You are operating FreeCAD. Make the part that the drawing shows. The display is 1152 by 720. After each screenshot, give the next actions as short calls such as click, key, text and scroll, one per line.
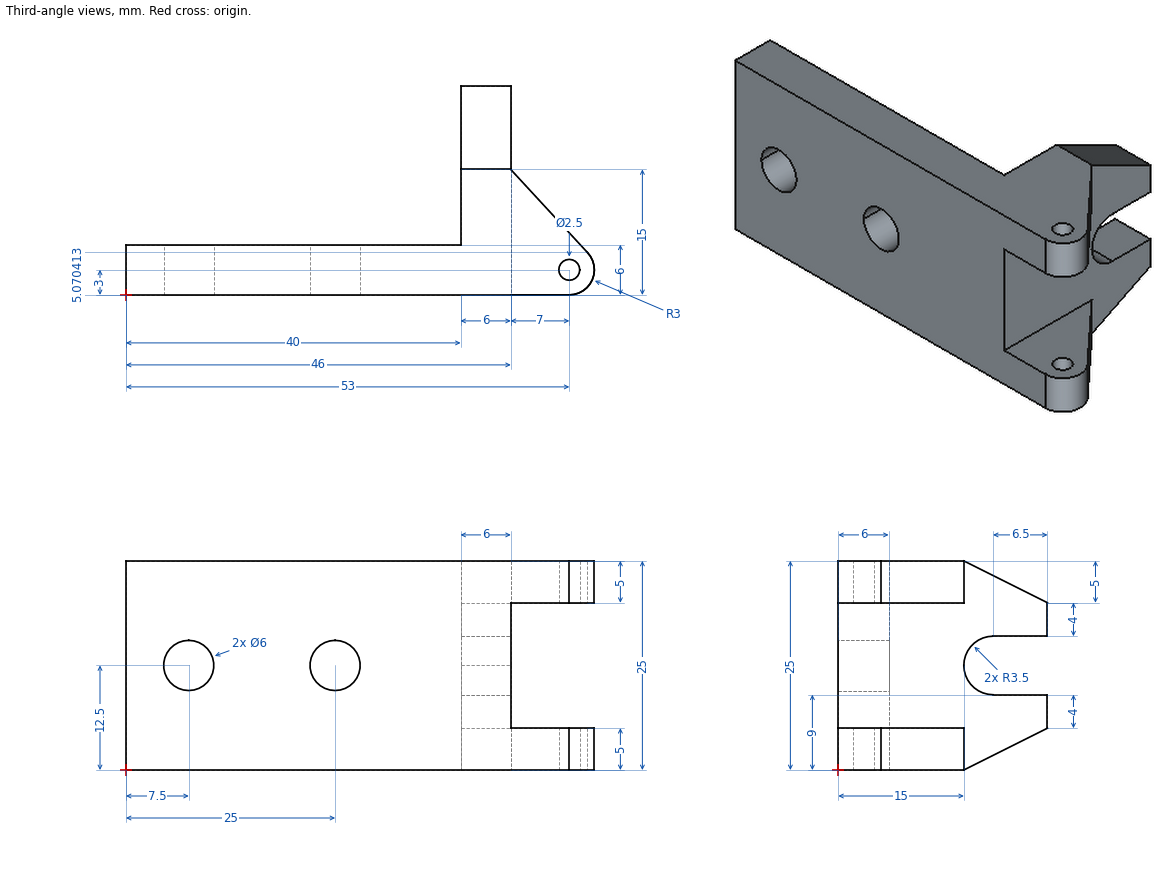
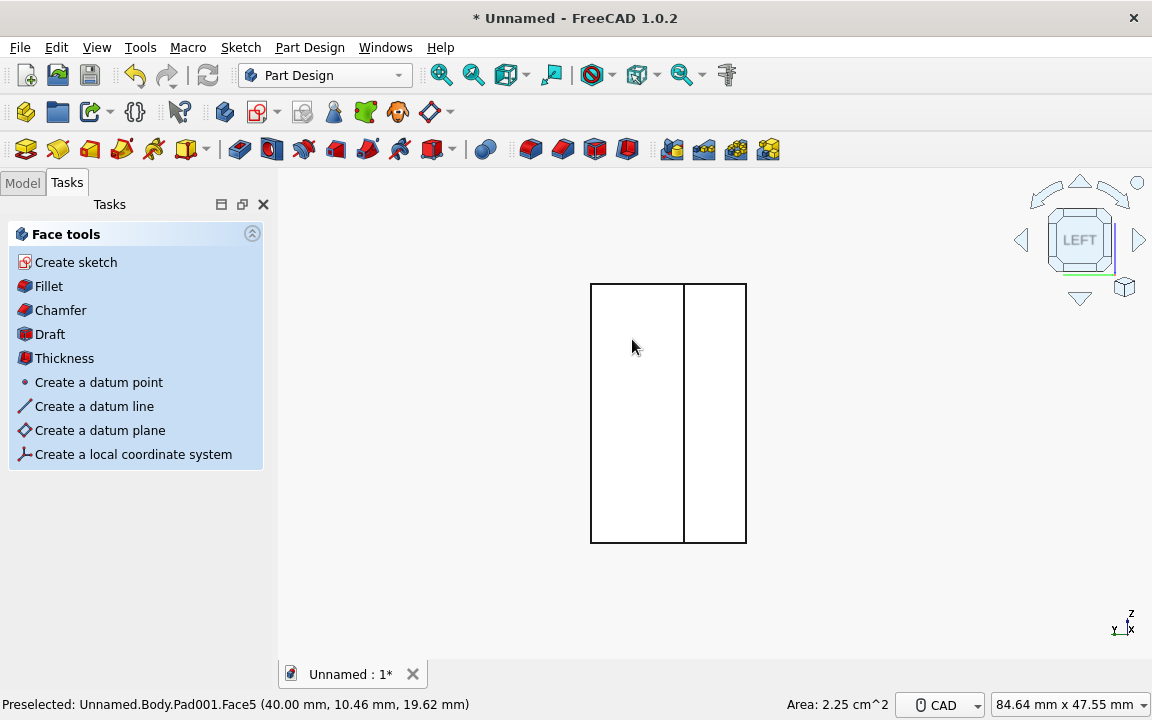
click(258, 112)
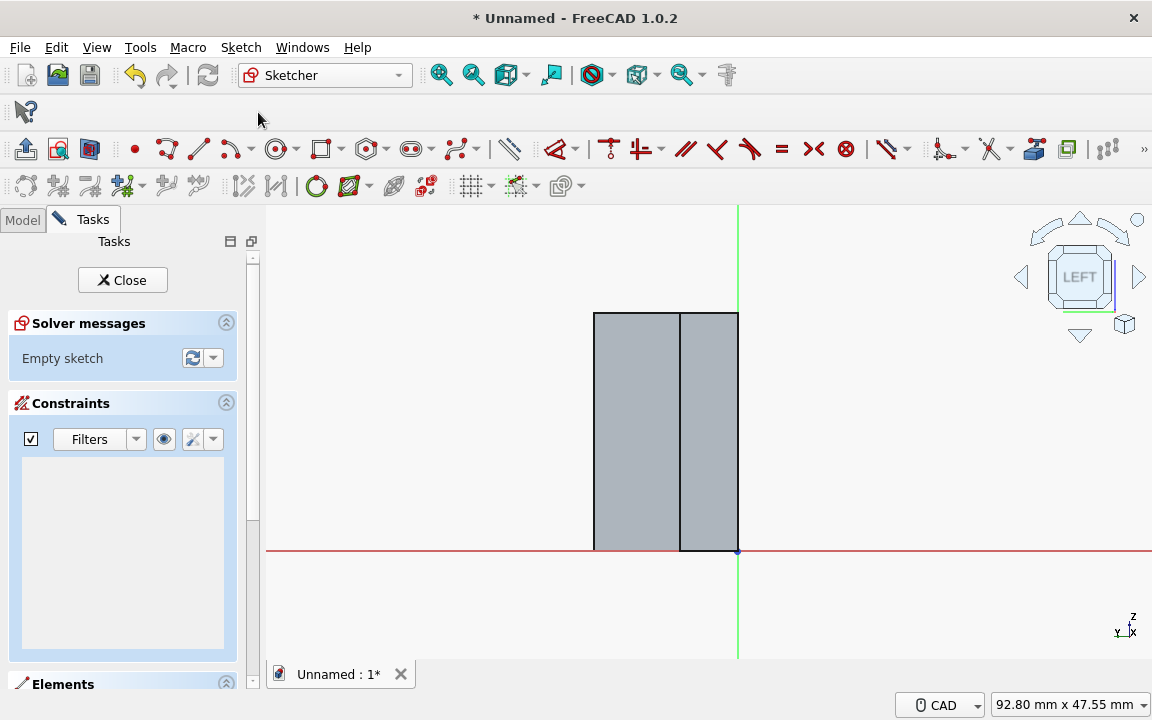
key(g)
key(m)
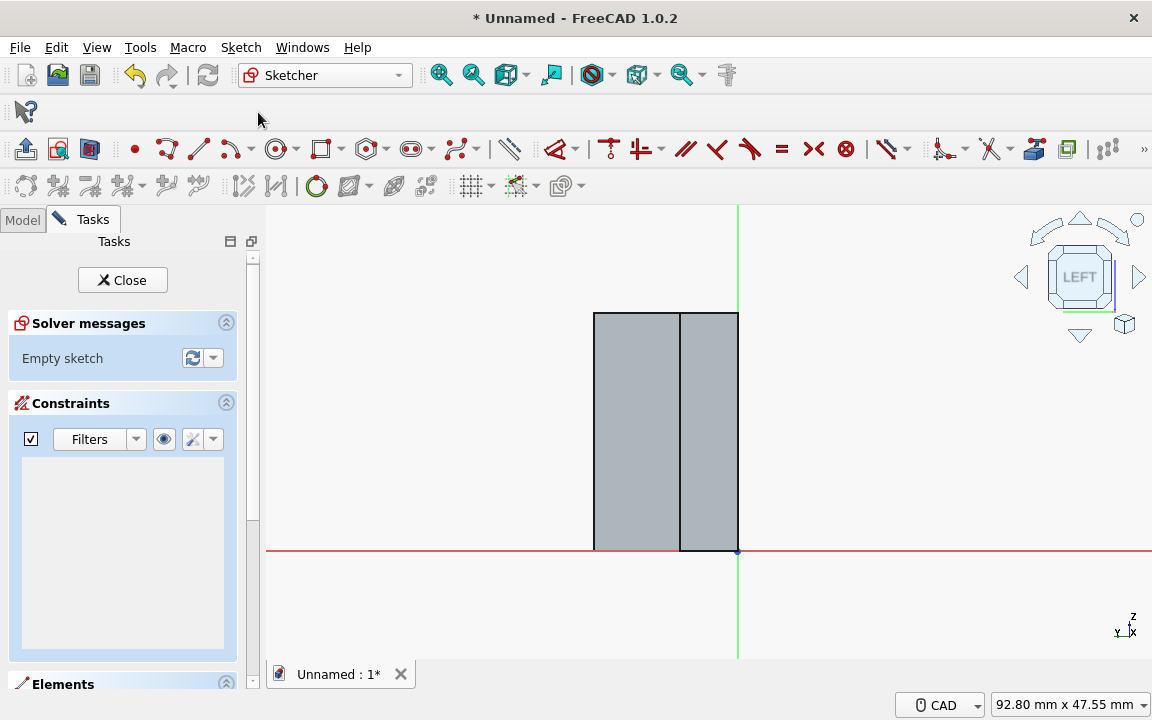
click(594, 432)
click(594, 313)
click(499, 360)
click(499, 399)
click(561, 399)
right_click(561, 399)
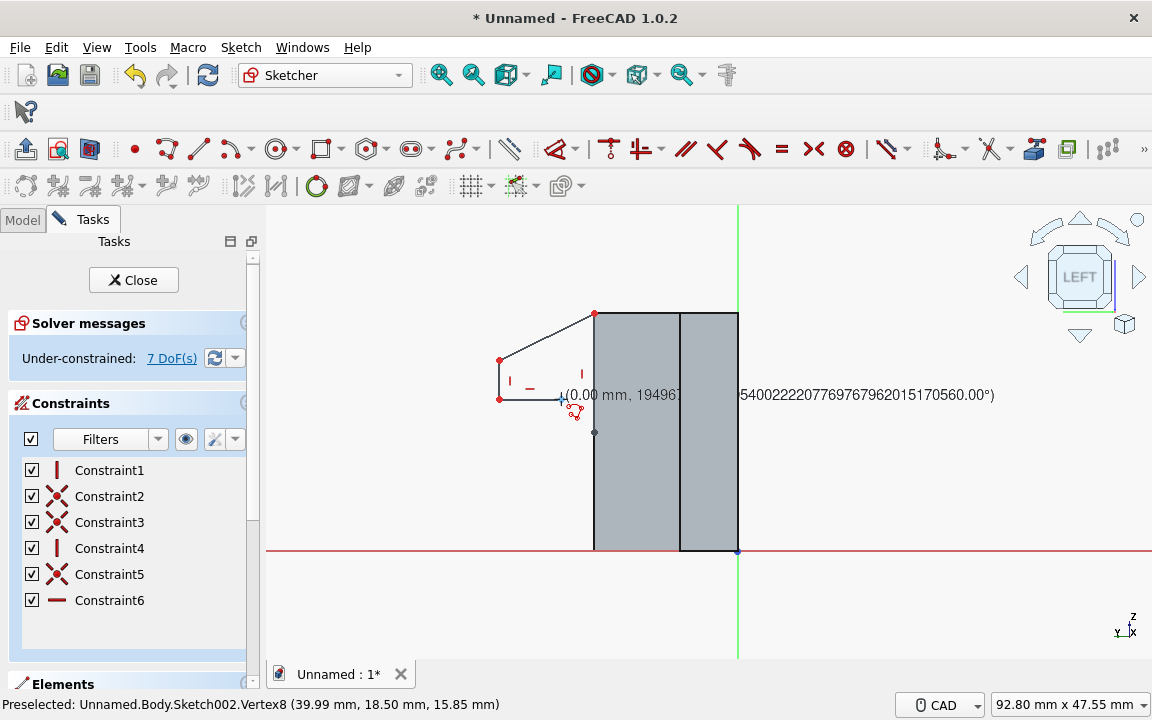
key(g)
key(3)
key(a)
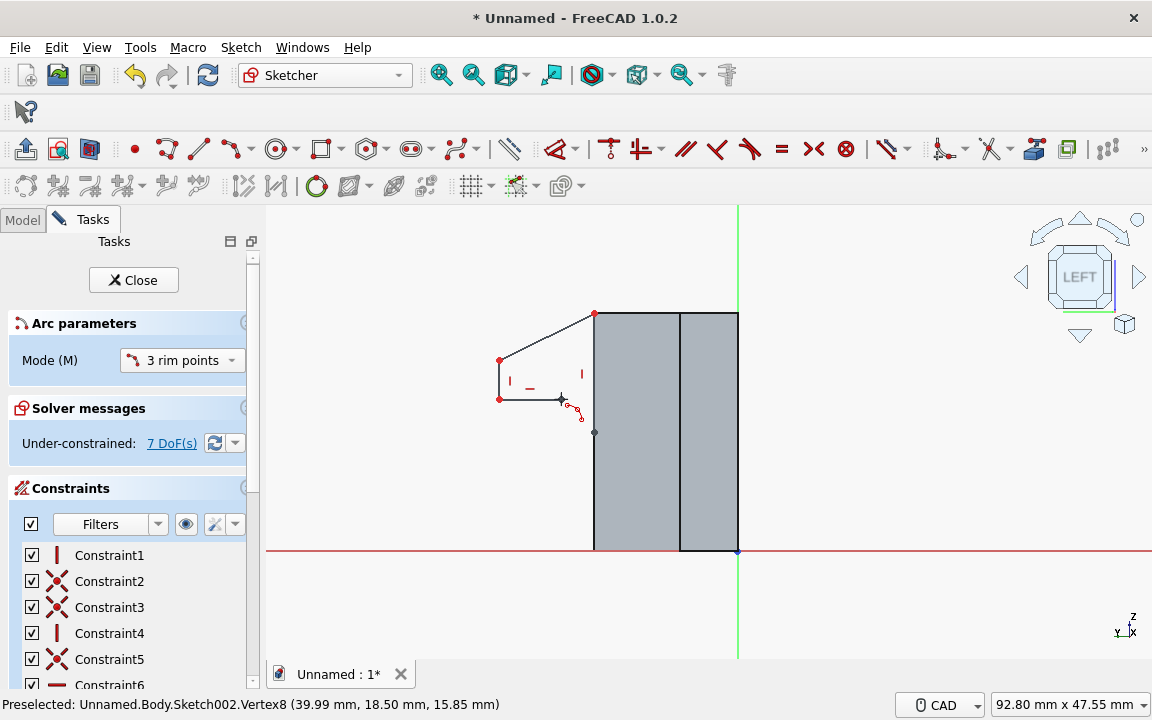
click(561, 400)
click(594, 433)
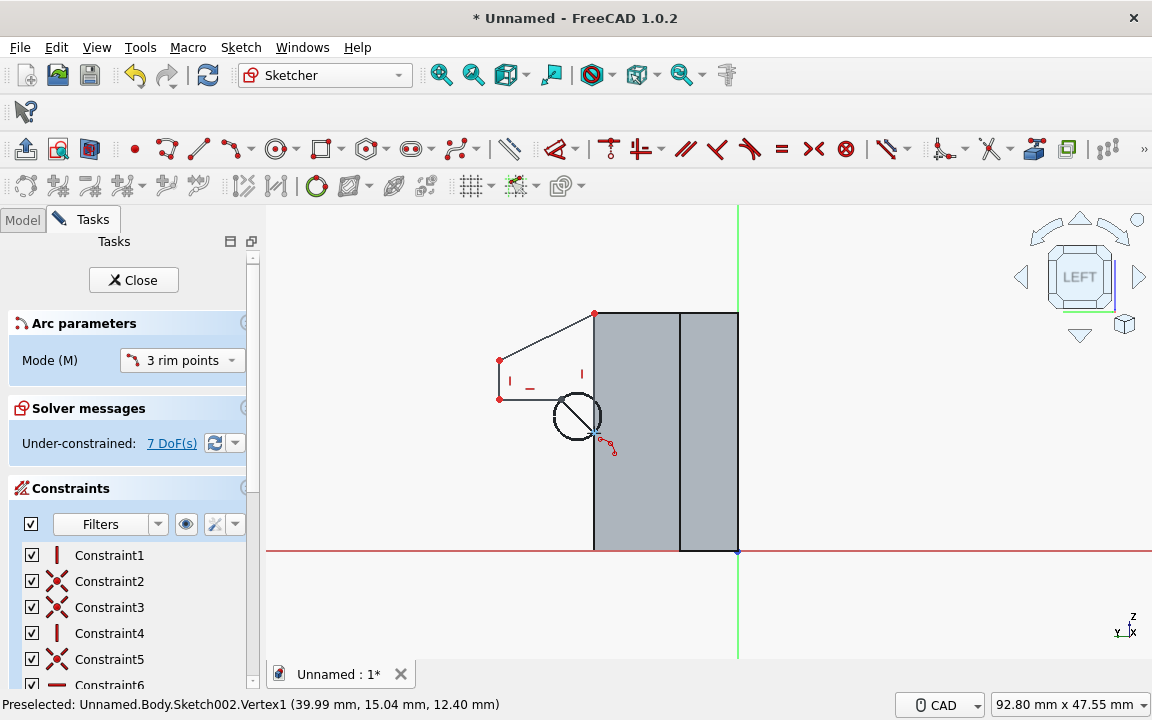
scroll(585, 408, up, 3)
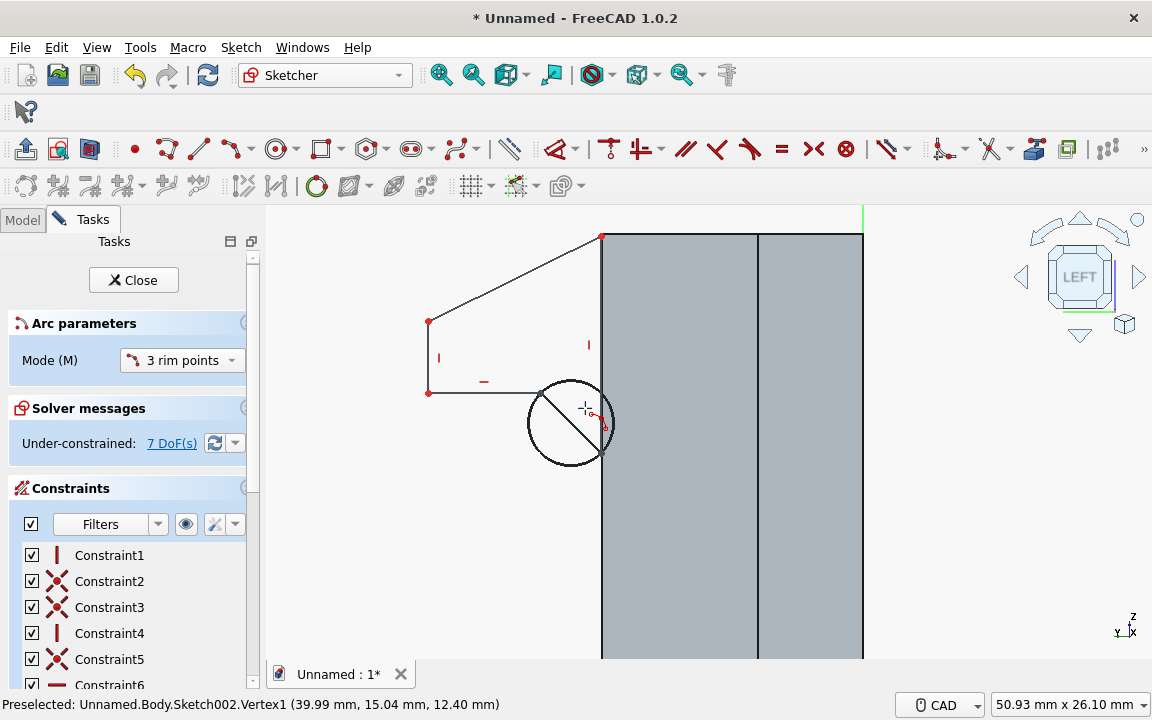
click(584, 408)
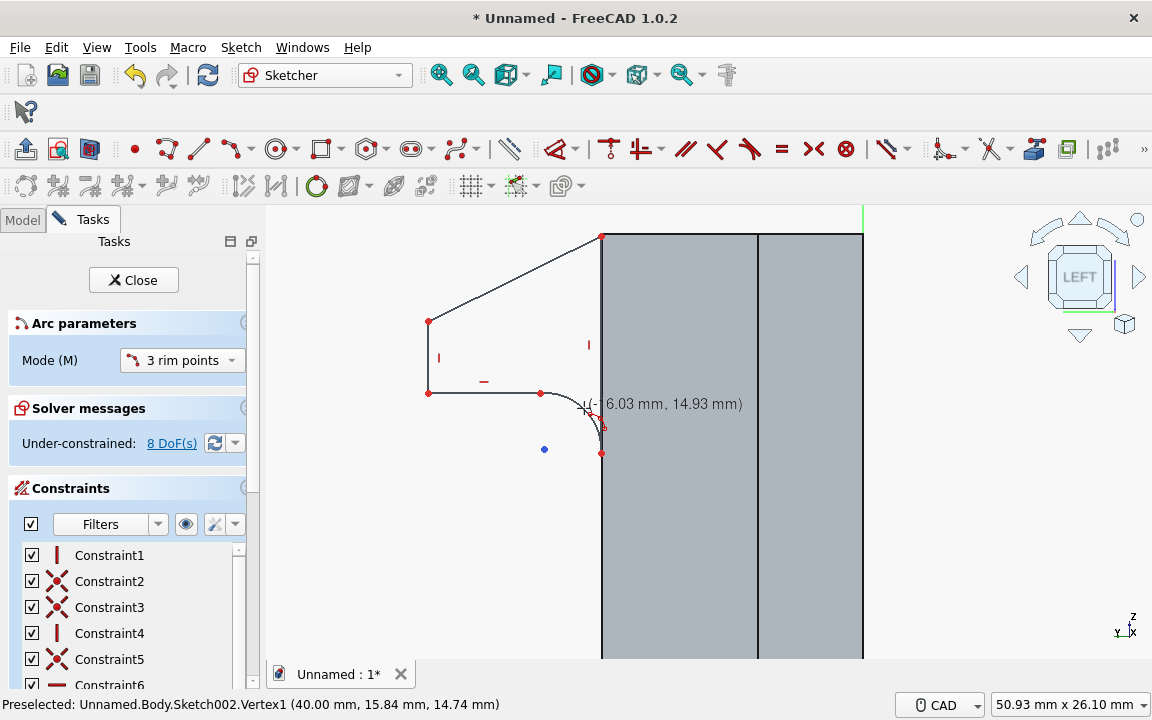
click(168, 150)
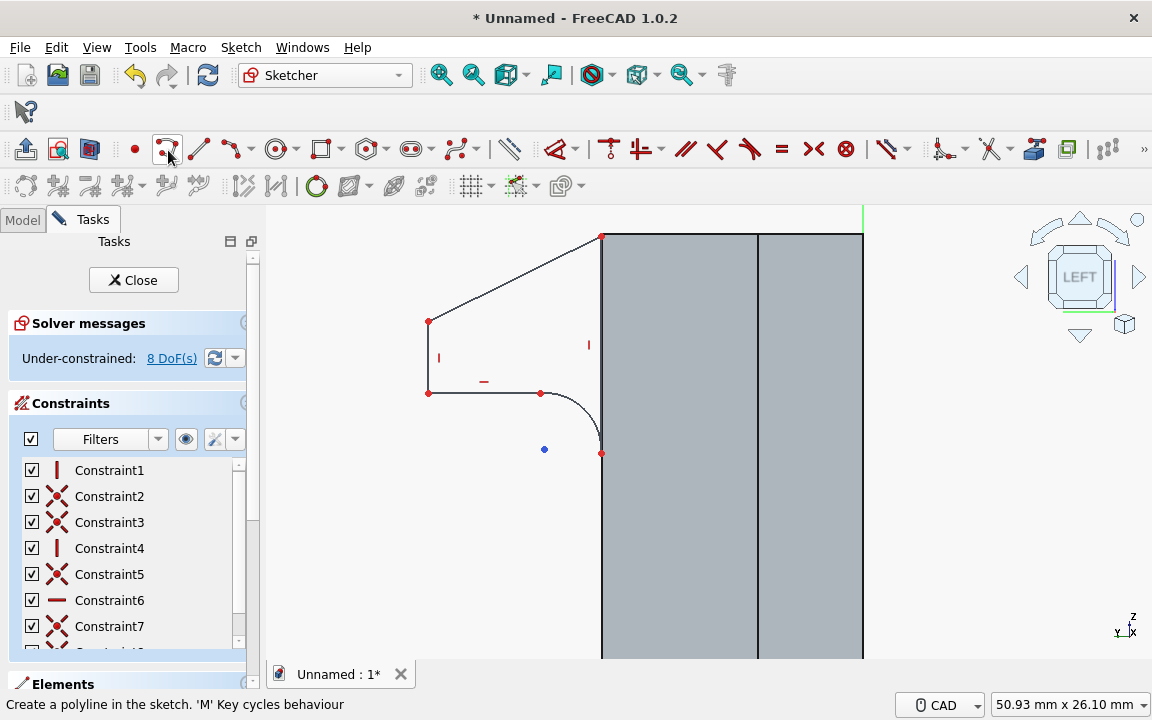
click(541, 512)
click(428, 512)
click(428, 582)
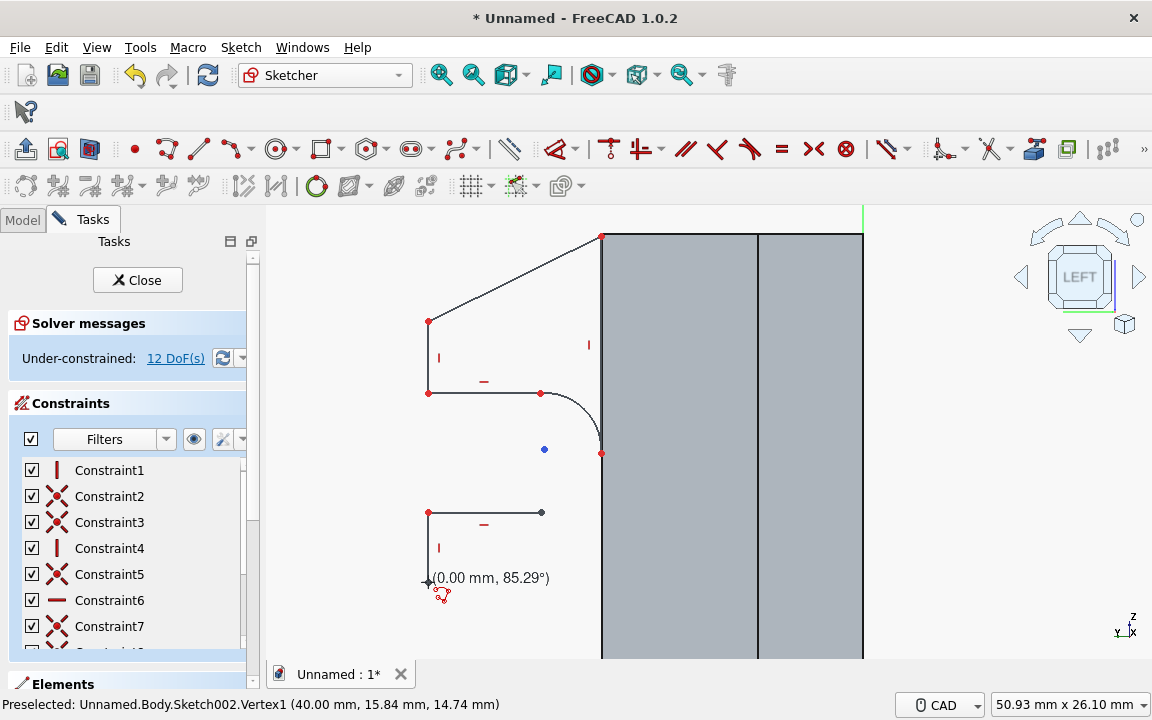
scroll(631, 393, down, 2)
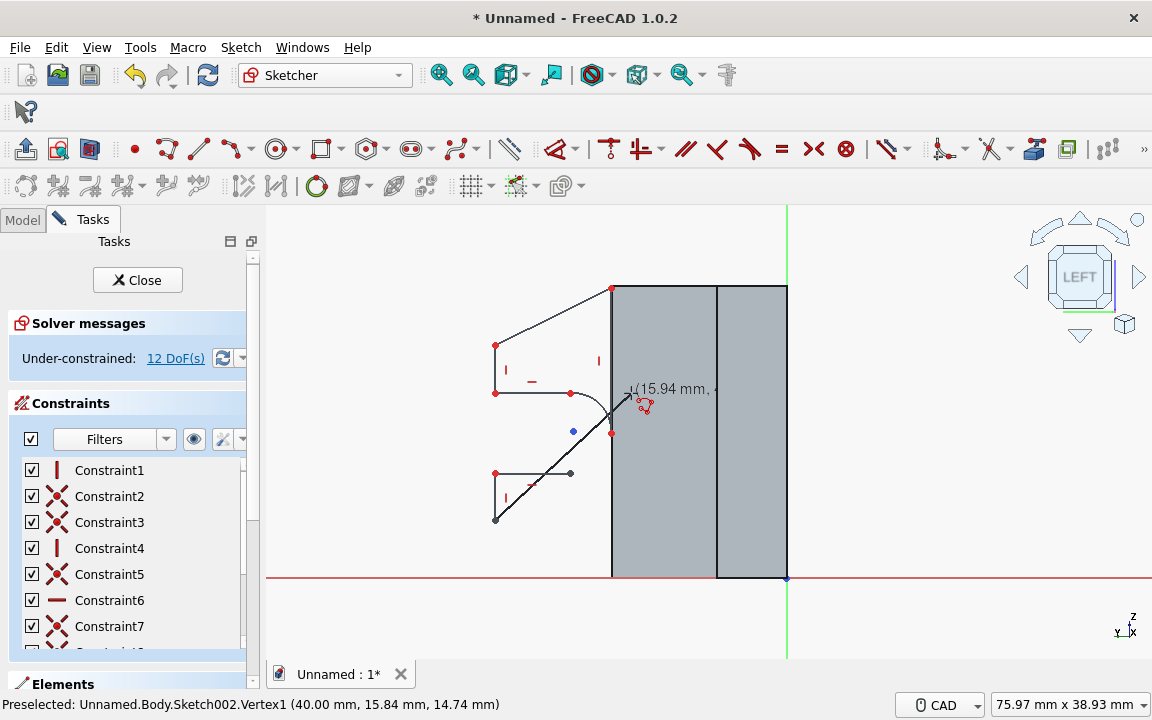
click(612, 578)
click(611, 433)
right_click(612, 578)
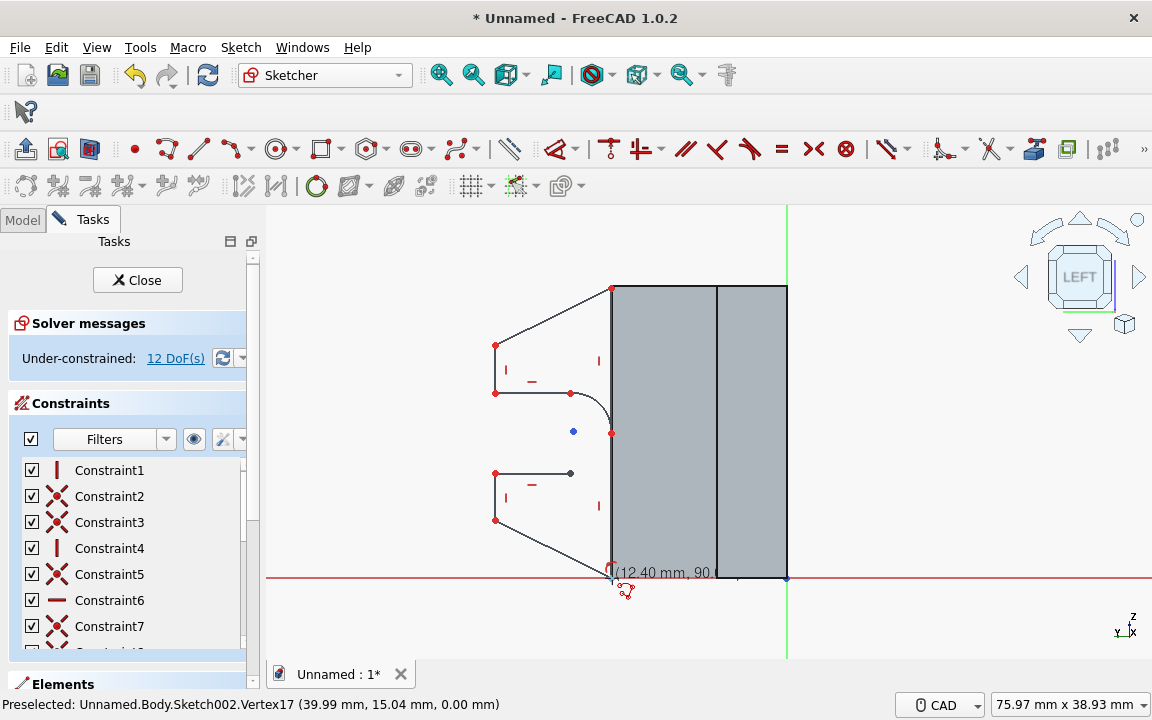
click(232, 150)